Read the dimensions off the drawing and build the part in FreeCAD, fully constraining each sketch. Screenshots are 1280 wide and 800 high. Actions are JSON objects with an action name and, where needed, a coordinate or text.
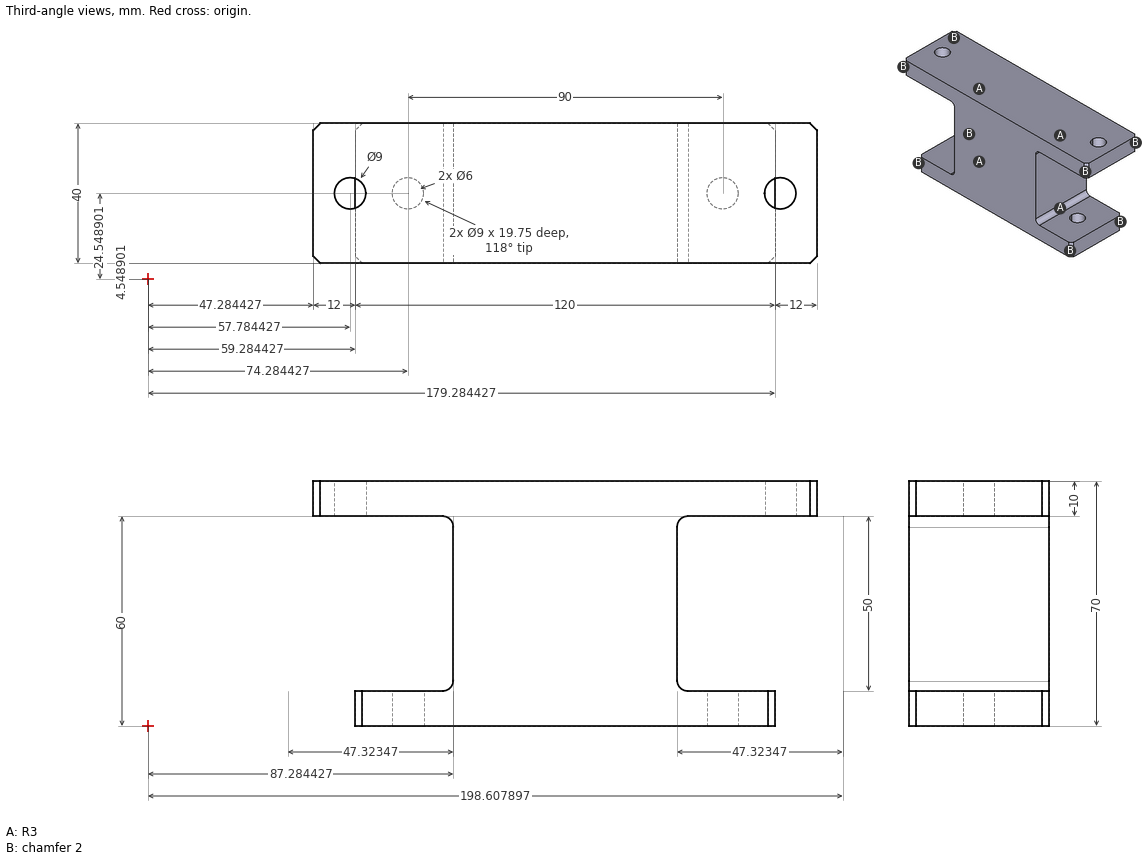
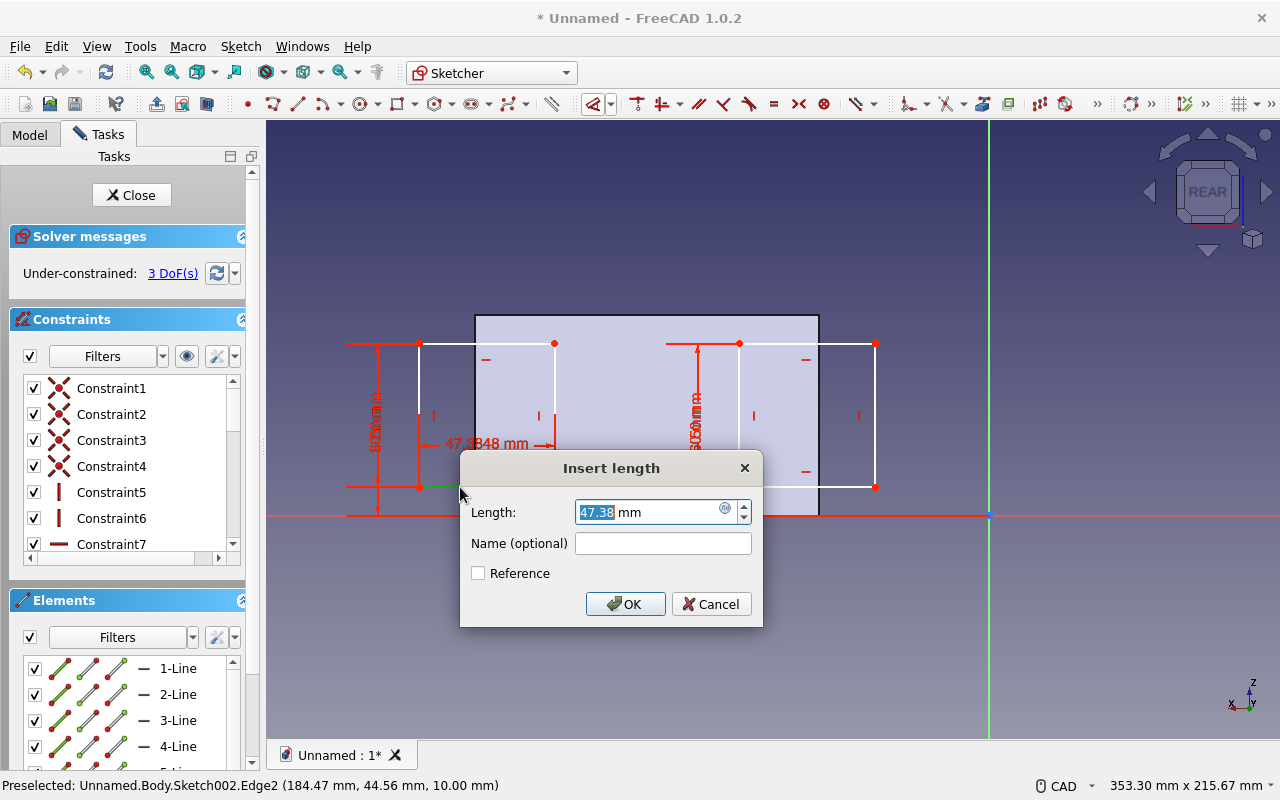
{"action": "type", "text": "47.32347"}
{"action": "key", "text": "Return"}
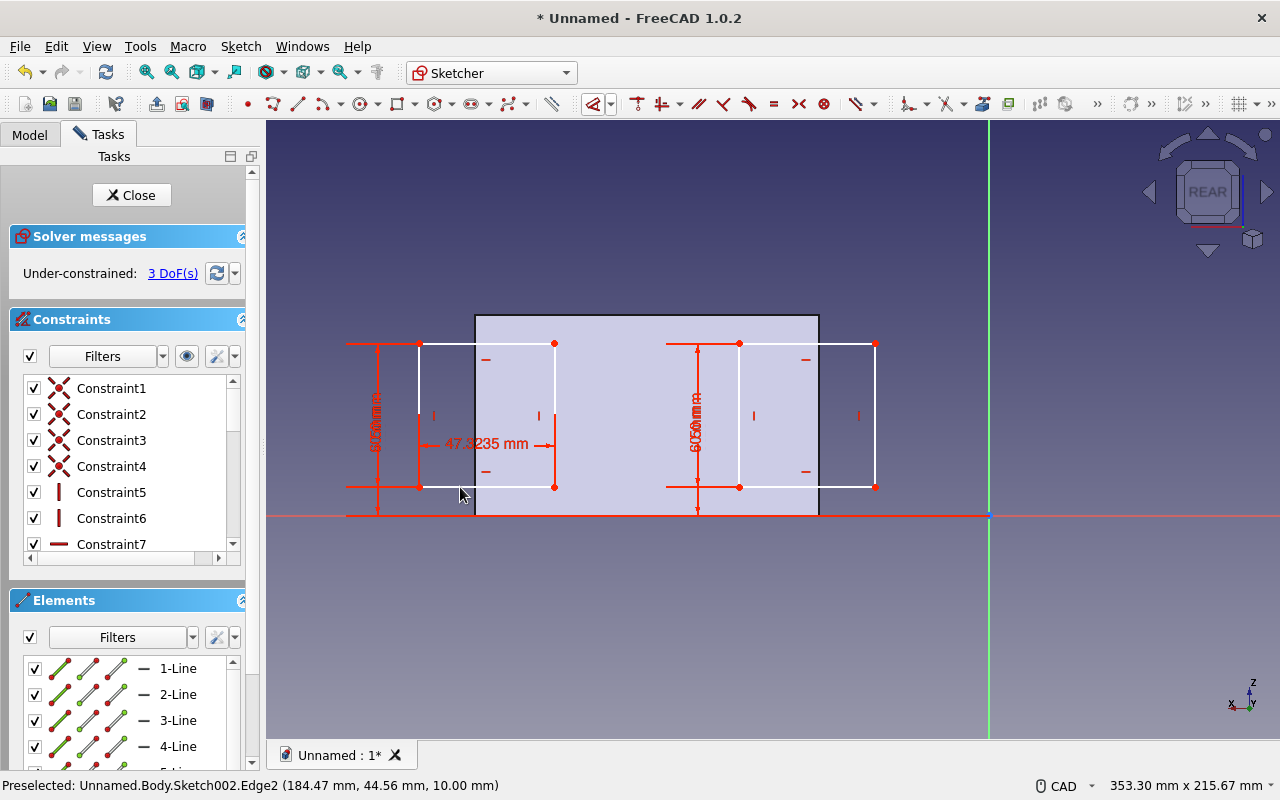
{"action": "left_click", "coordinate": [780, 487]}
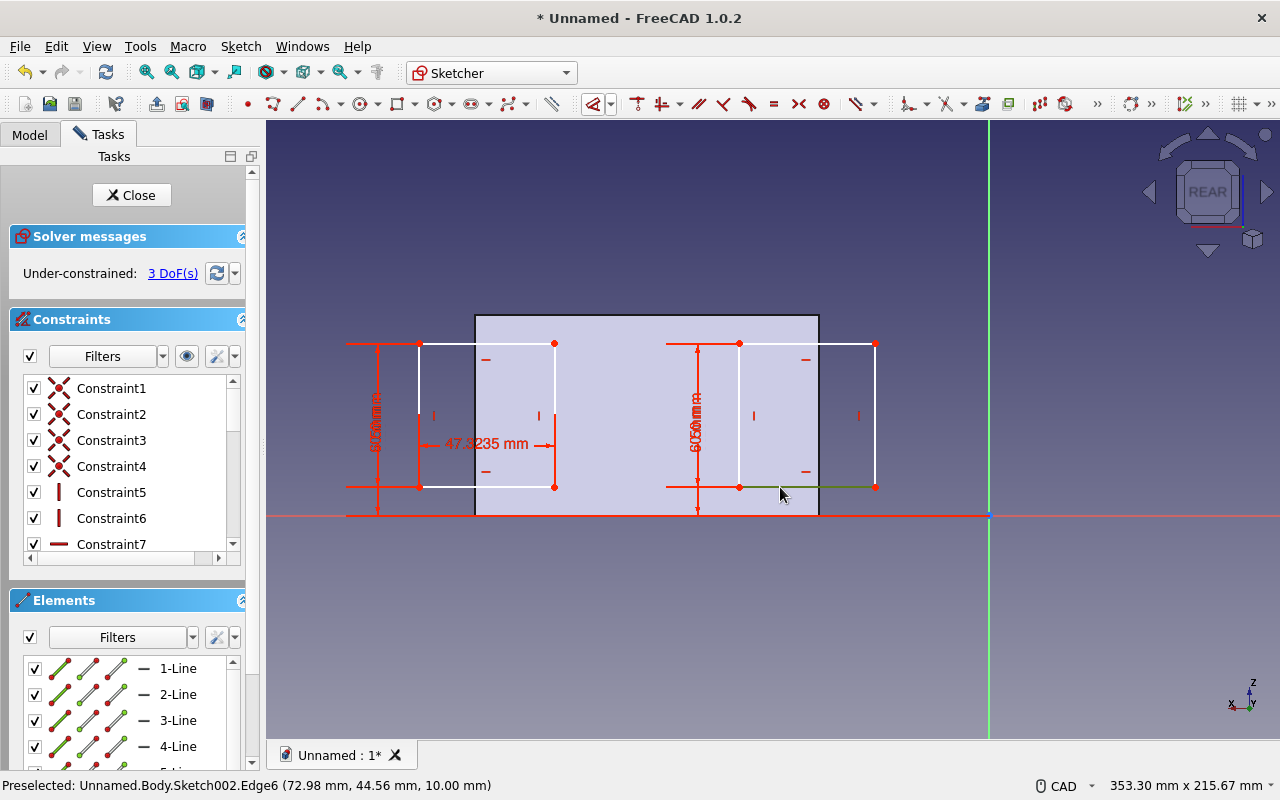
{"action": "key", "text": "l"}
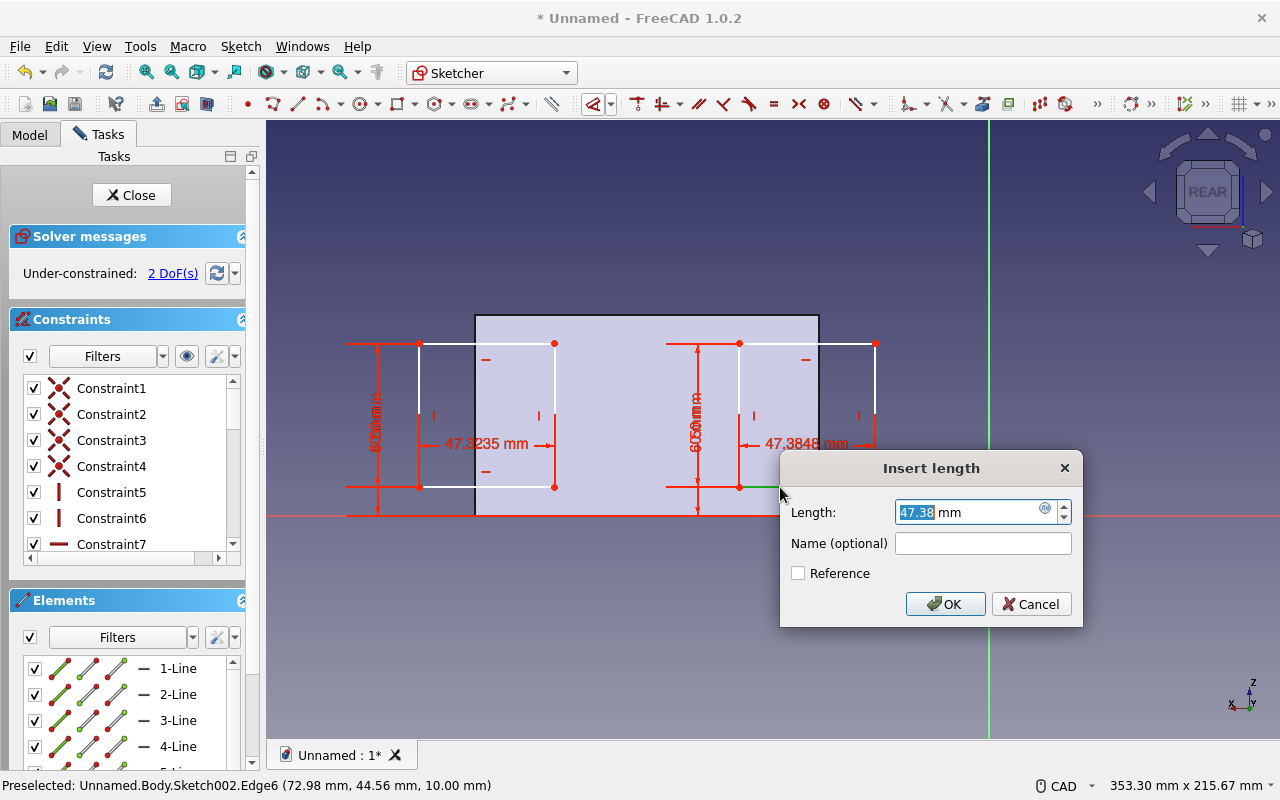
{"action": "type", "text": "47.32347"}
{"action": "key", "text": "Return"}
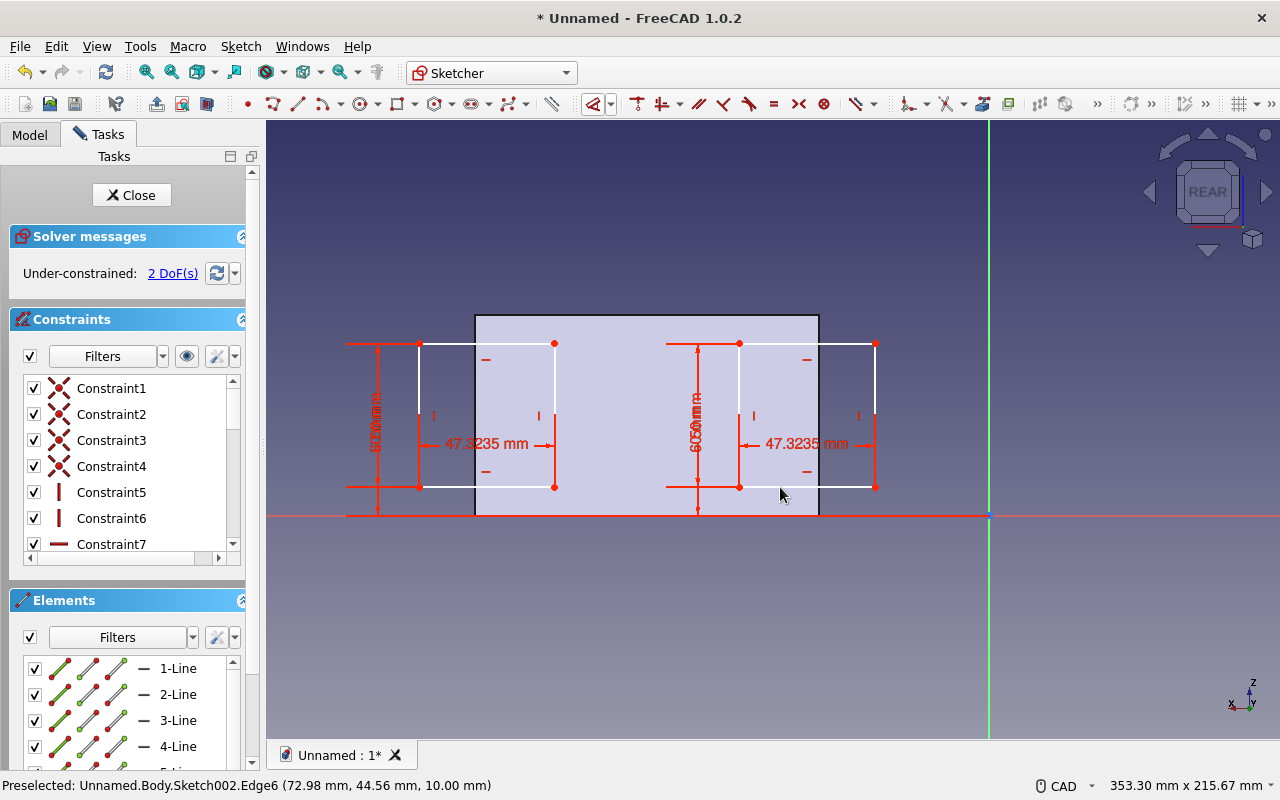
{"action": "left_click", "coordinate": [739, 344]}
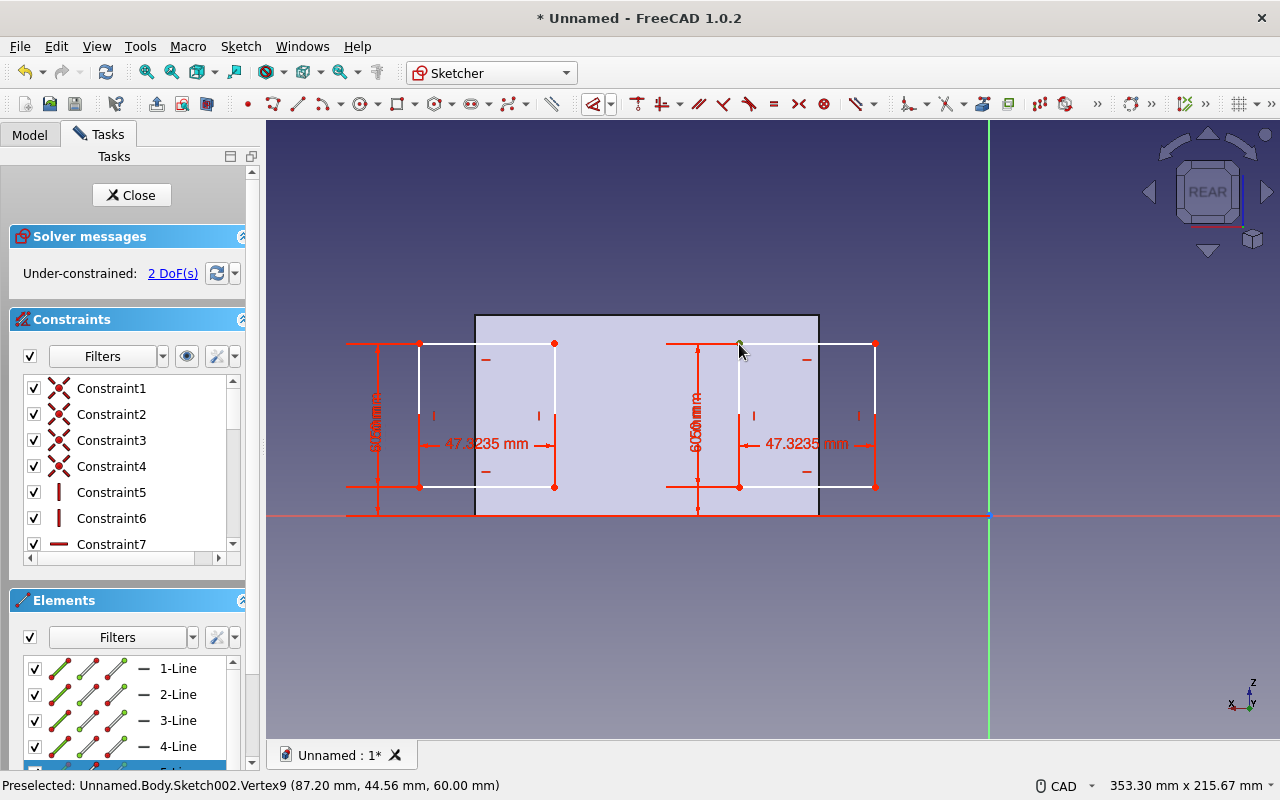
{"action": "key", "text": "l"}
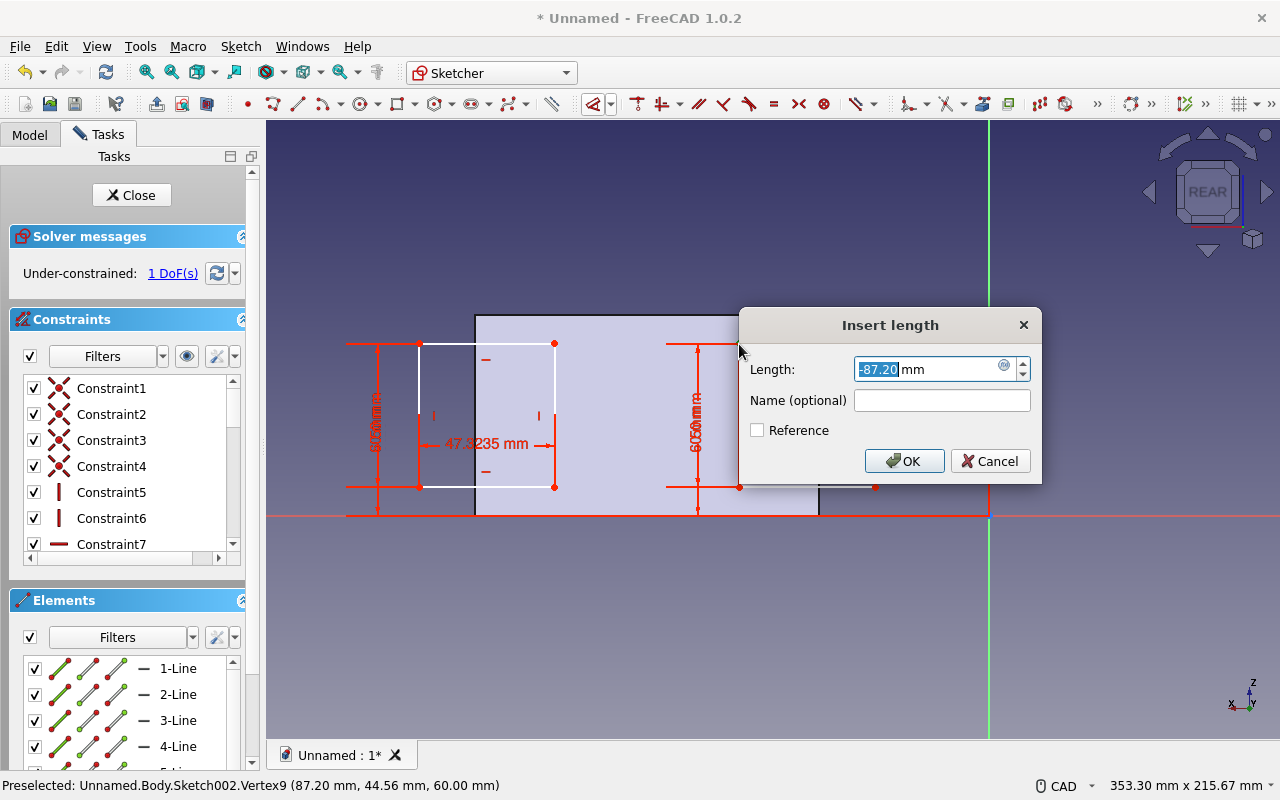
{"action": "type", "text": "-87.284427"}
{"action": "key", "text": "Return"}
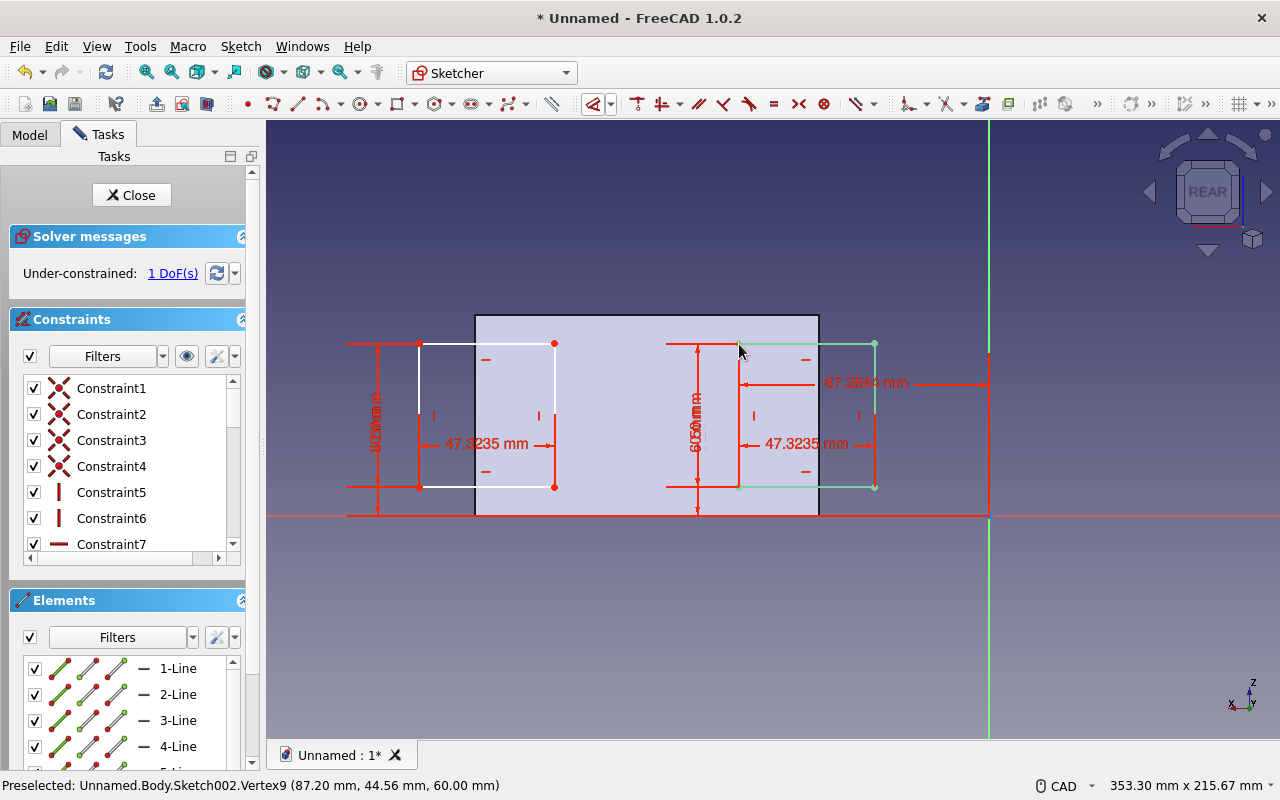
{"action": "left_click", "coordinate": [419, 344]}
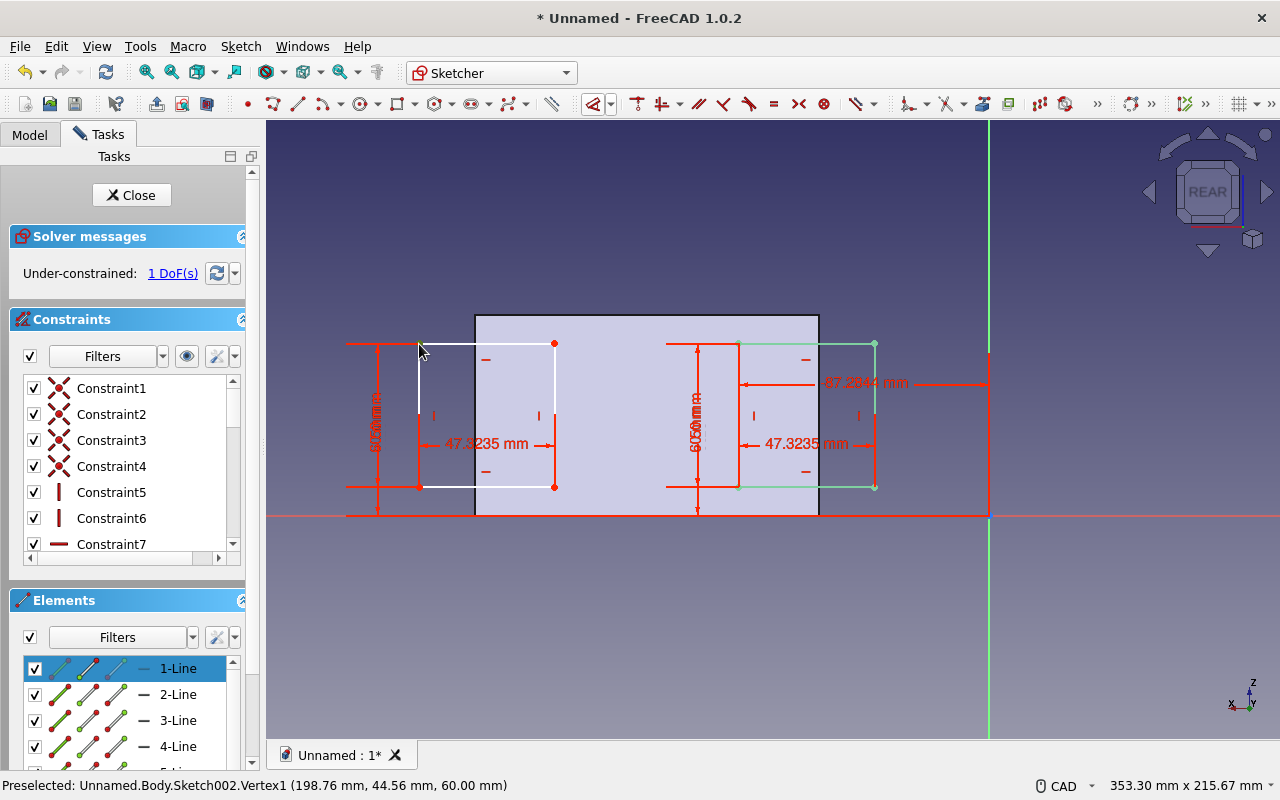
{"action": "key", "text": "l"}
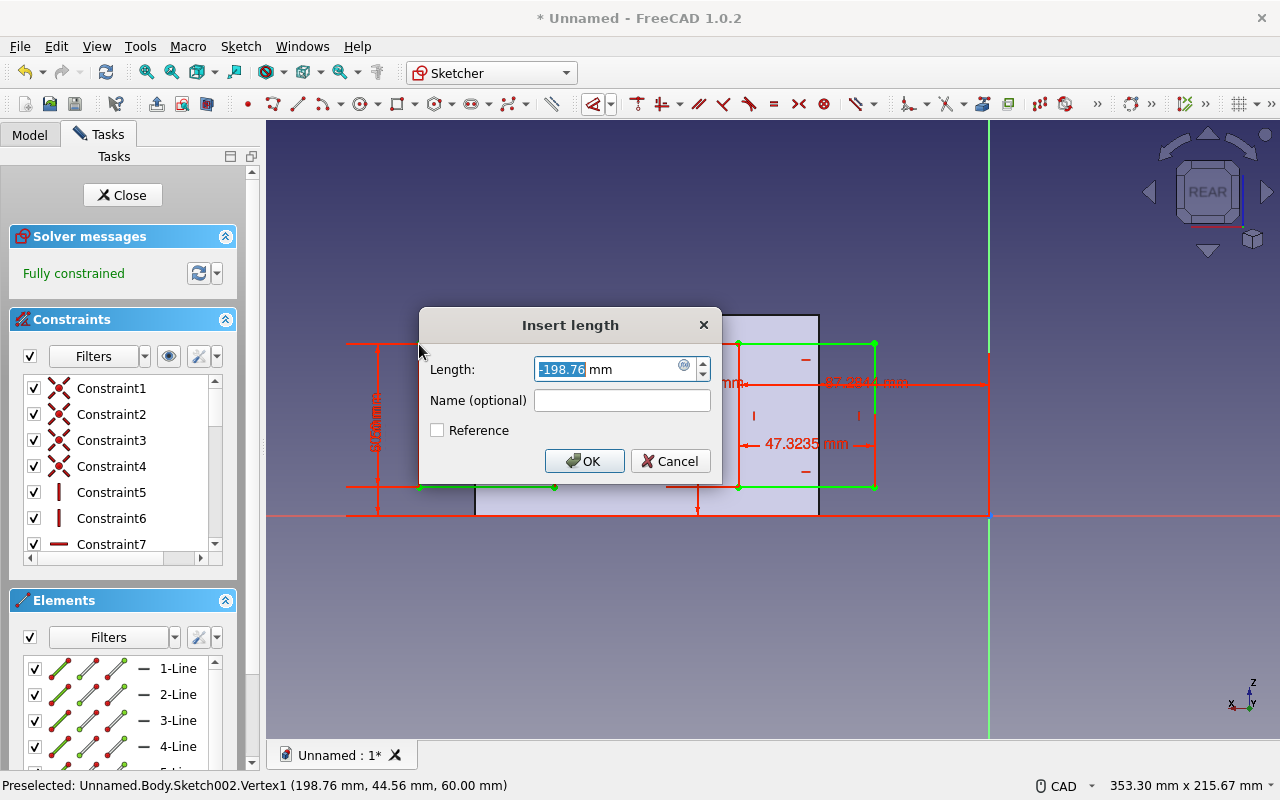
{"action": "type", "text": "-198.607897"}
{"action": "key", "text": "Return"}